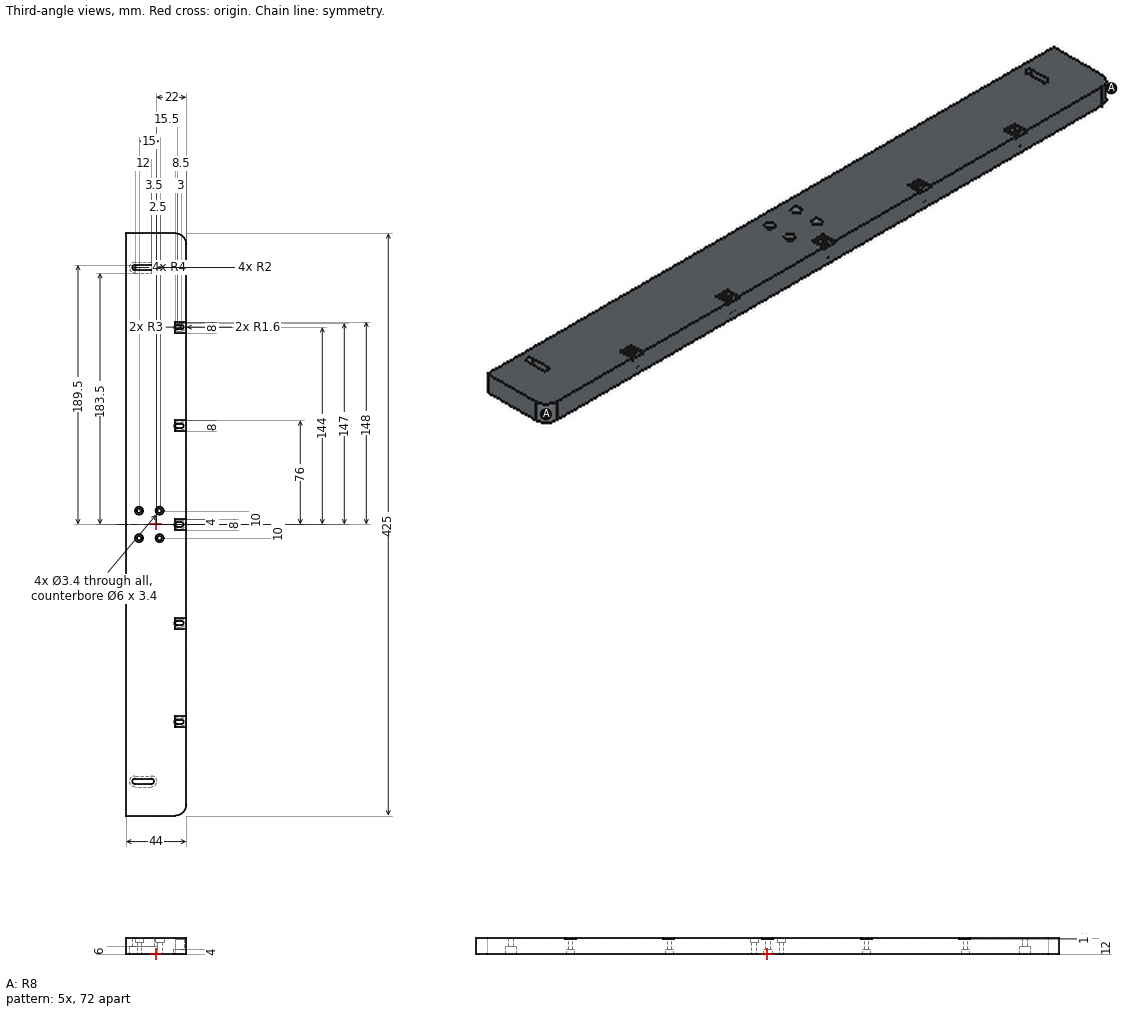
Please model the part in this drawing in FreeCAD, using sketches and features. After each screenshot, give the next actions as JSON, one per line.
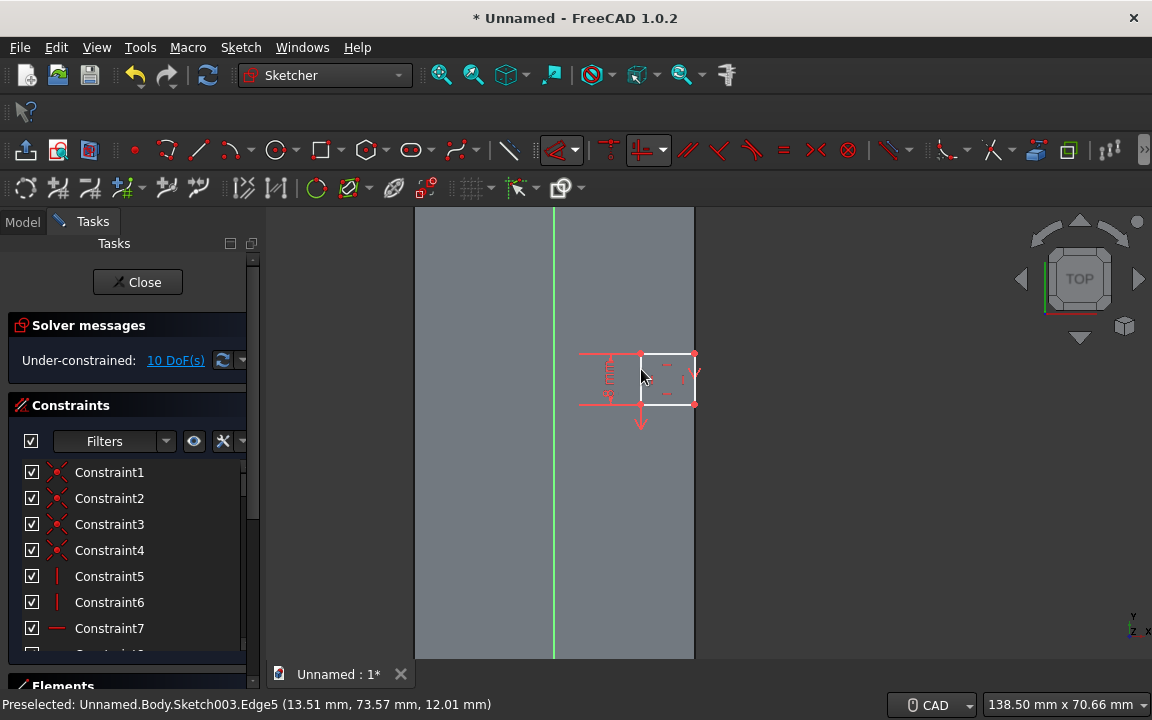
{"action": "scroll", "coordinate": [643, 369], "scroll_direction": "down", "scroll_amount": 10}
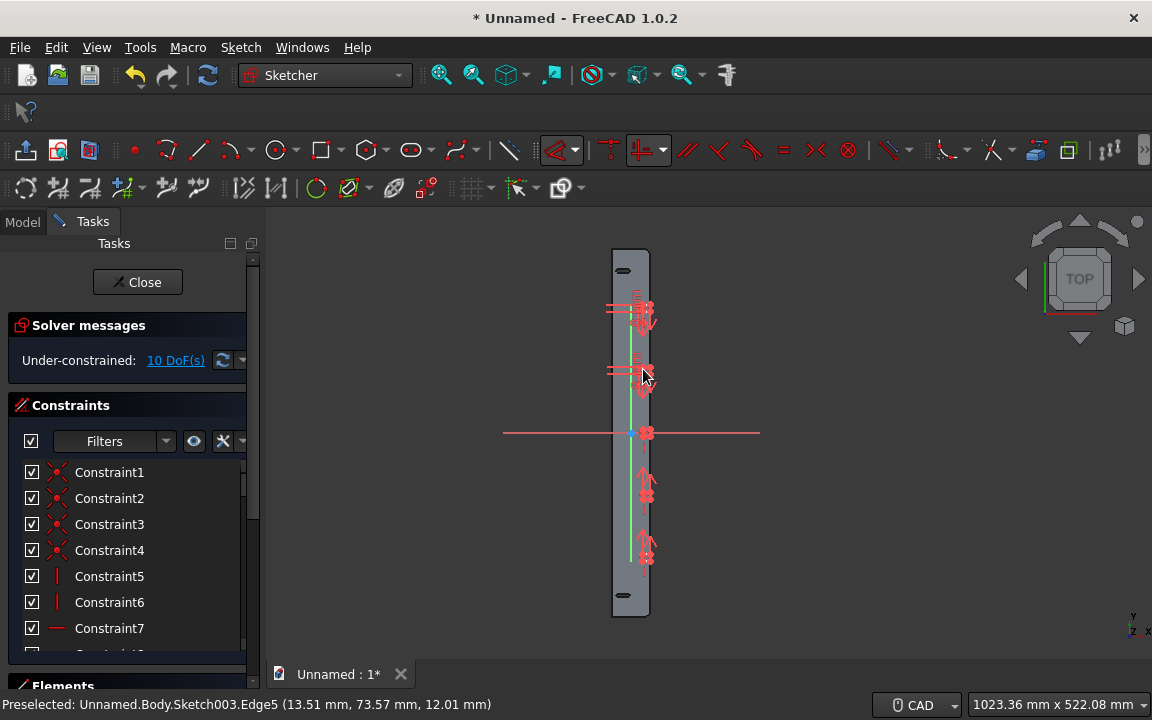
{"action": "scroll", "coordinate": [643, 435], "scroll_direction": "up", "scroll_amount": 11}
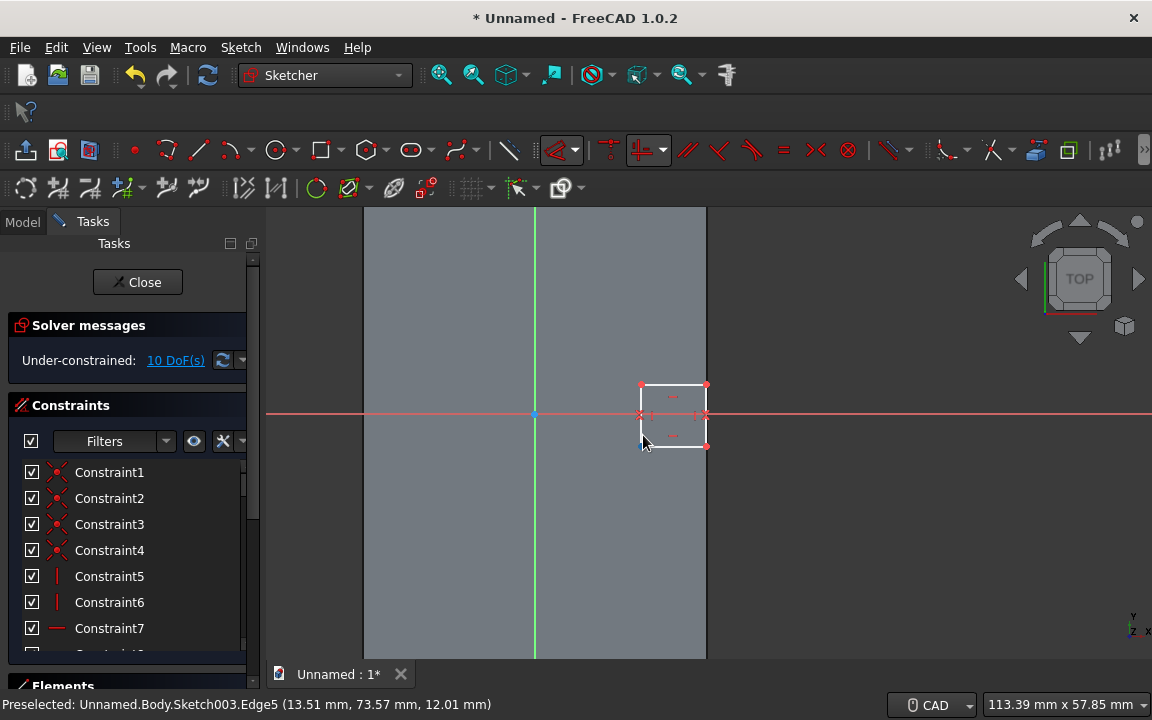
{"action": "left_click", "coordinate": [641, 428]}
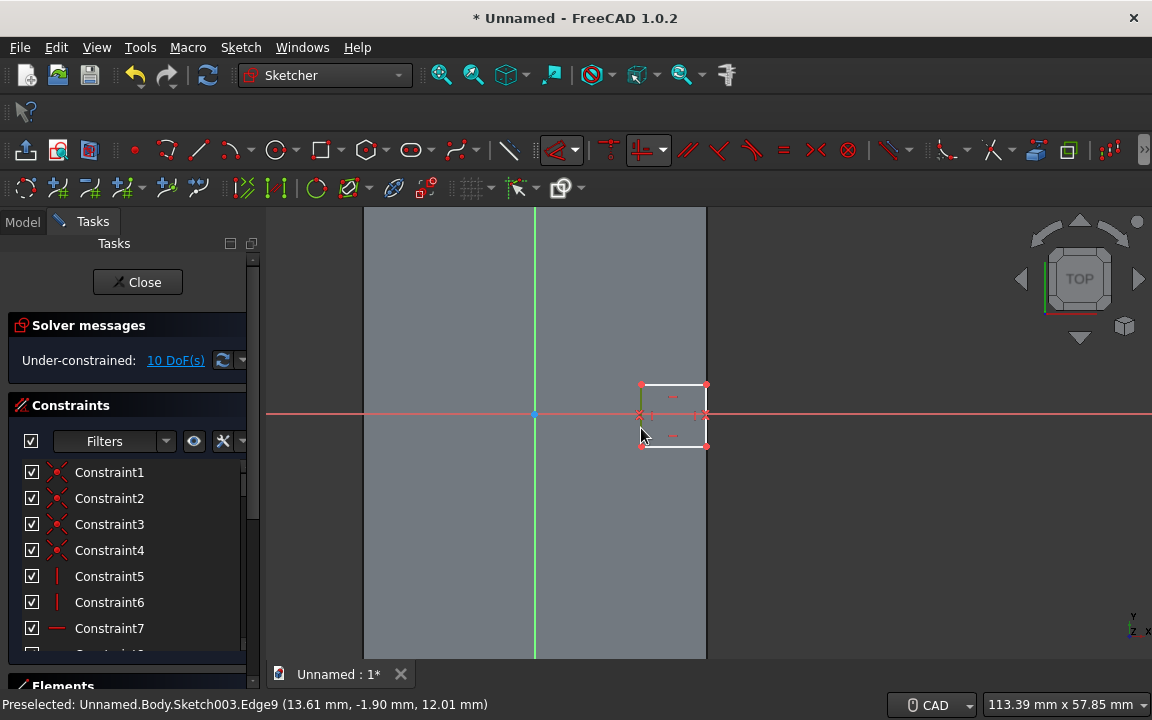
{"action": "key", "text": "i"}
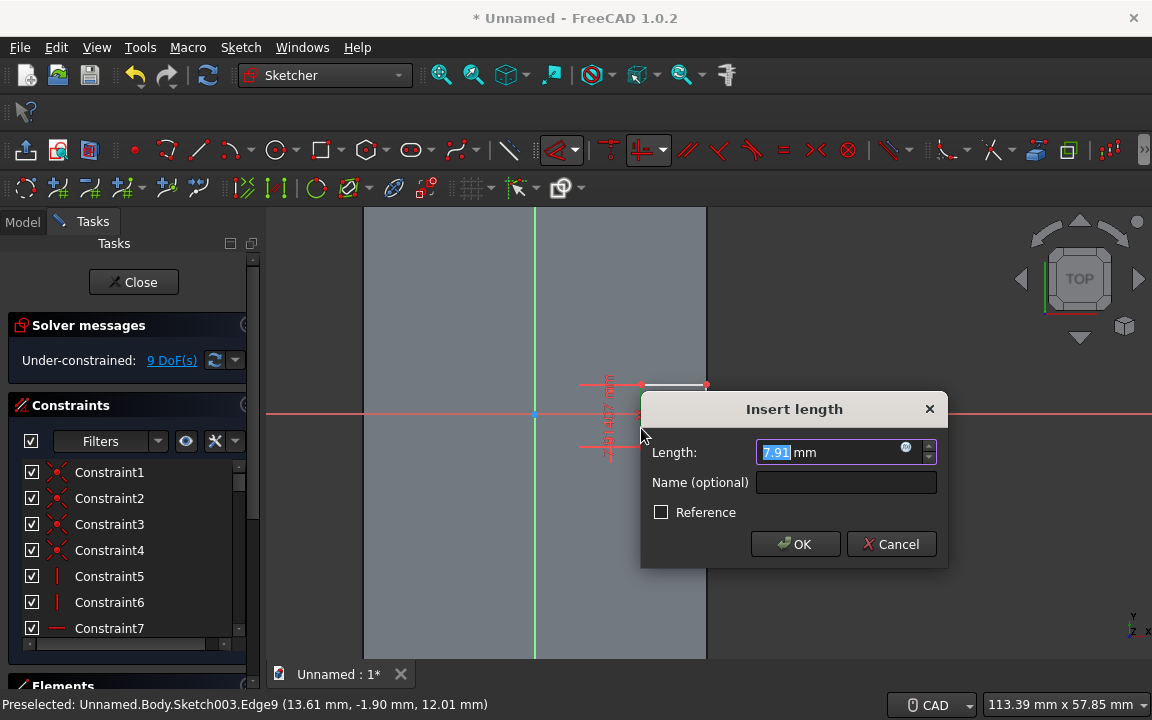
{"action": "type", "text": "8"}
{"action": "key", "text": "Return"}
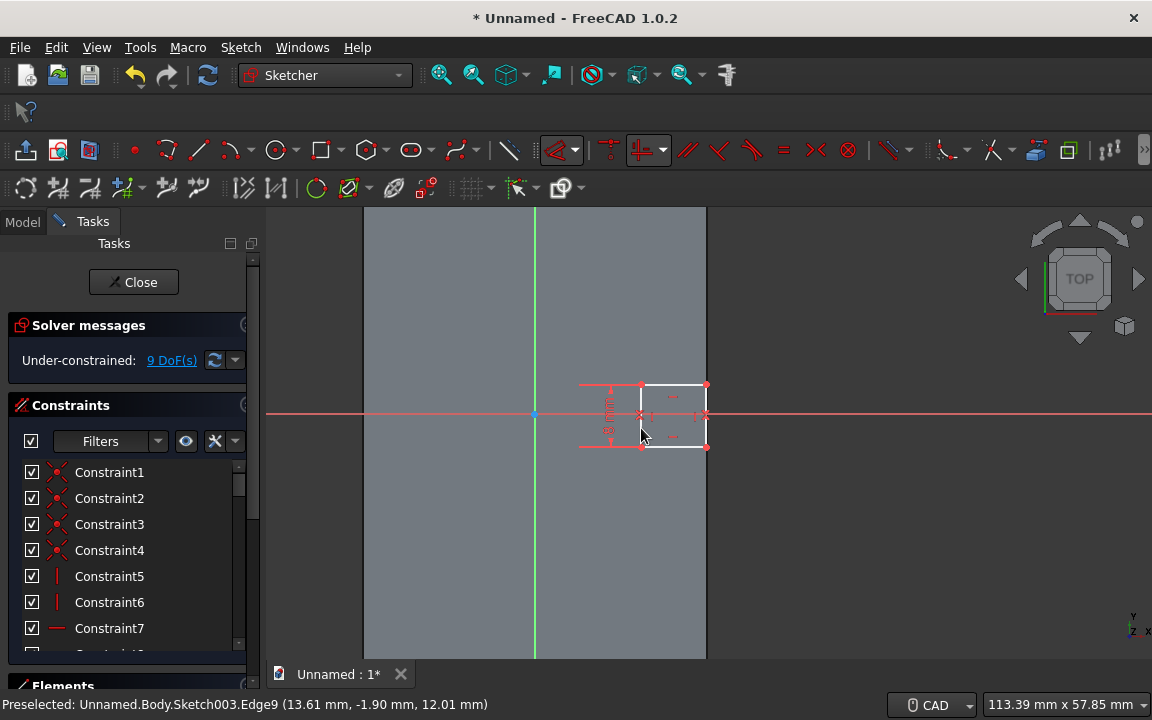
{"action": "scroll", "coordinate": [641, 385], "scroll_direction": "up", "scroll_amount": 2}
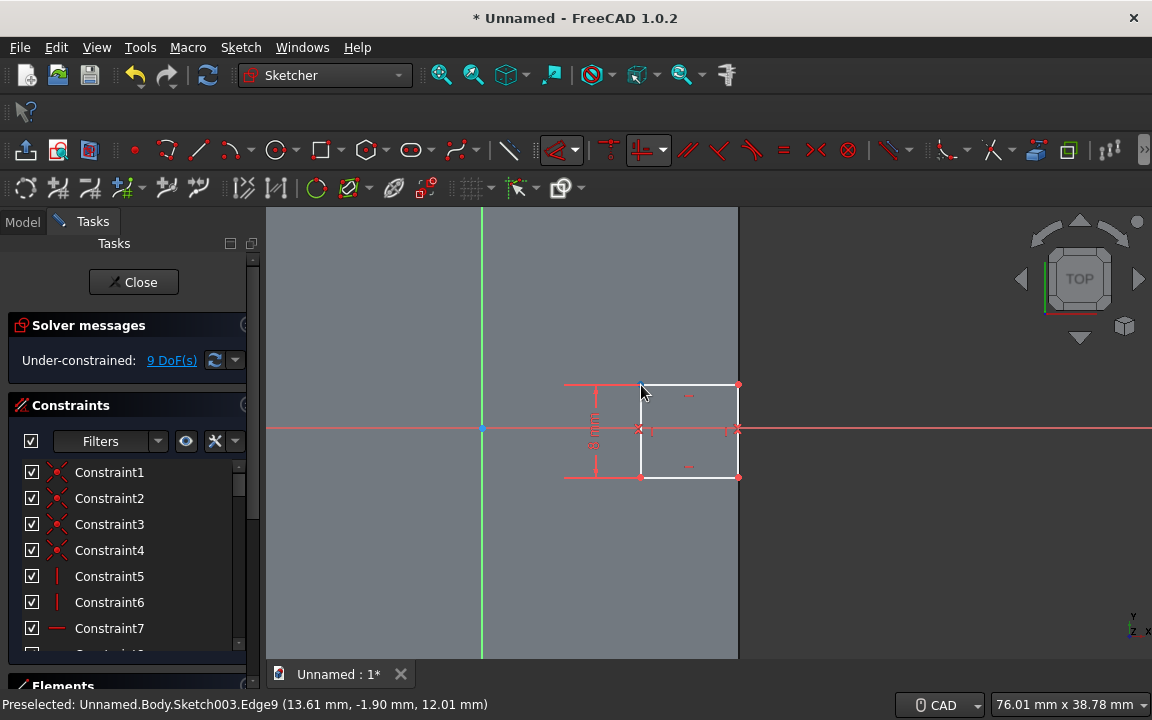
{"action": "left_click", "coordinate": [641, 385]}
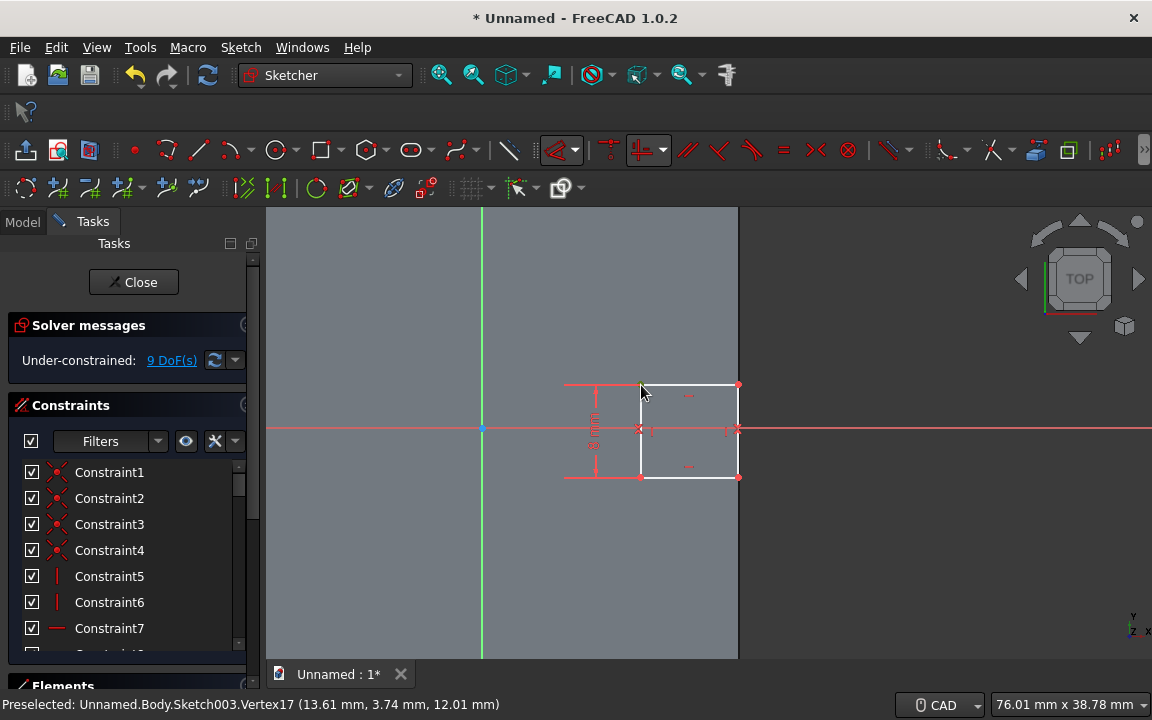
{"action": "key", "text": "i"}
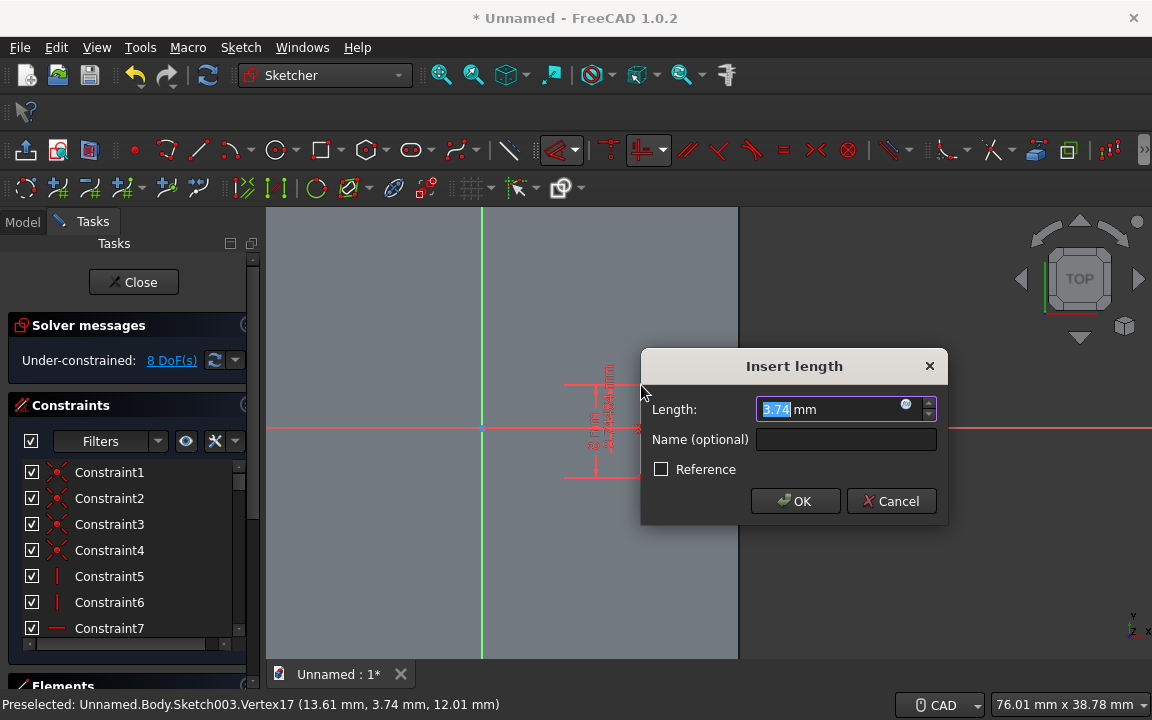
{"action": "type", "text": "4"}
{"action": "key", "text": "Return"}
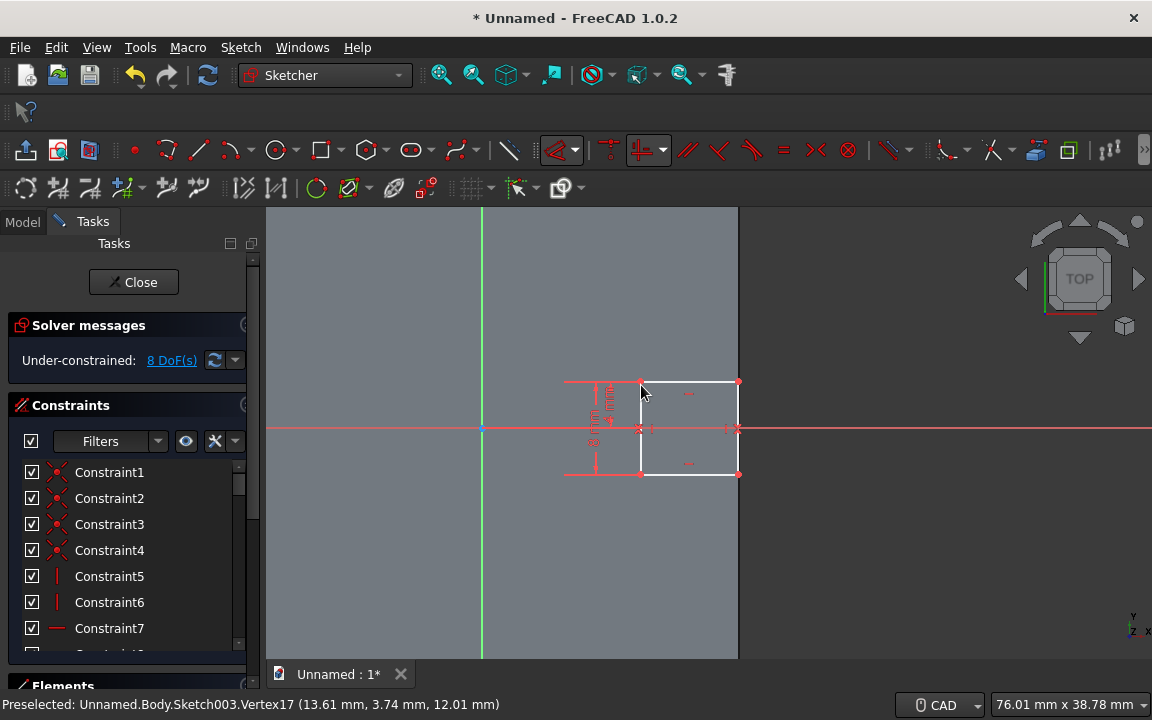
{"action": "scroll", "coordinate": [643, 433], "scroll_direction": "down", "scroll_amount": 13}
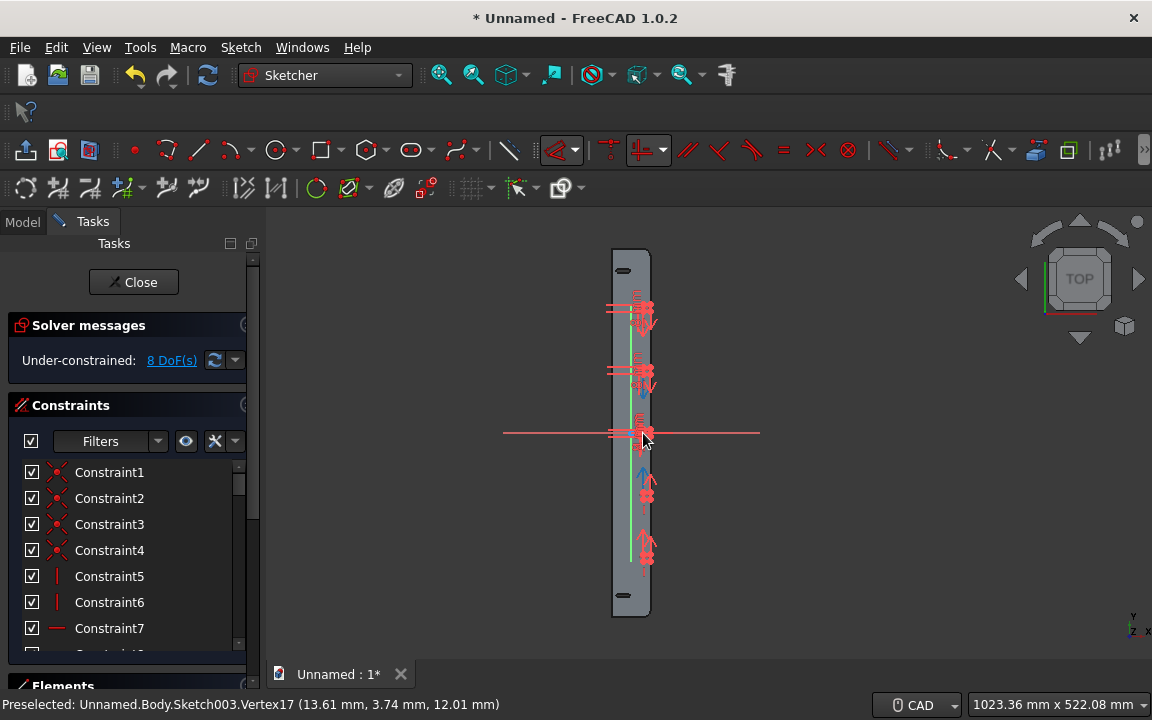
{"action": "scroll", "coordinate": [645, 312], "scroll_direction": "up", "scroll_amount": 10}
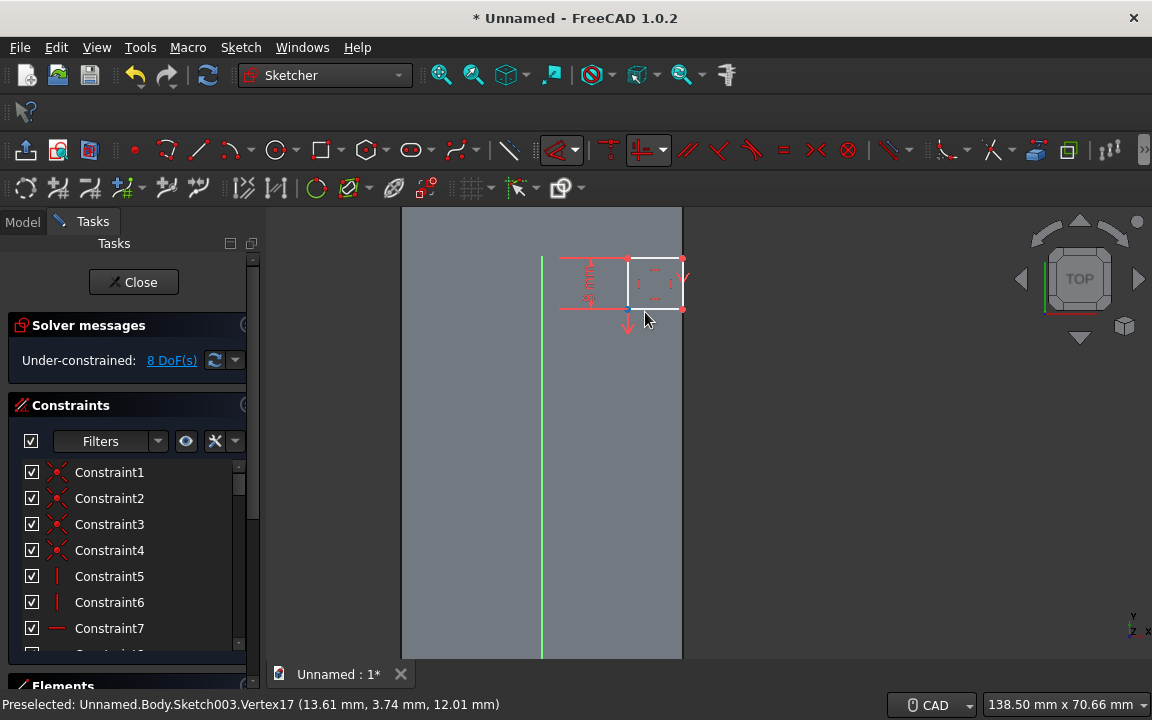
{"action": "left_click", "coordinate": [644, 309]}